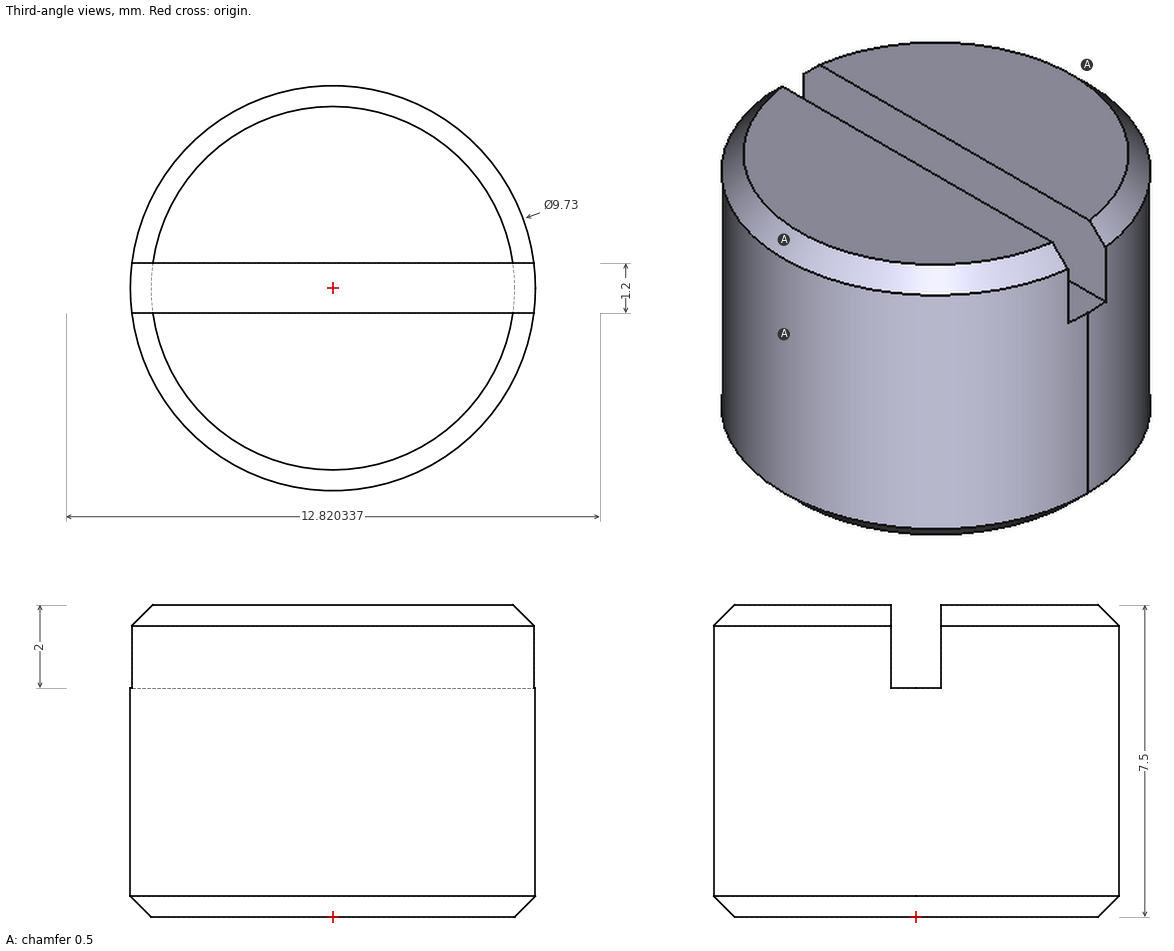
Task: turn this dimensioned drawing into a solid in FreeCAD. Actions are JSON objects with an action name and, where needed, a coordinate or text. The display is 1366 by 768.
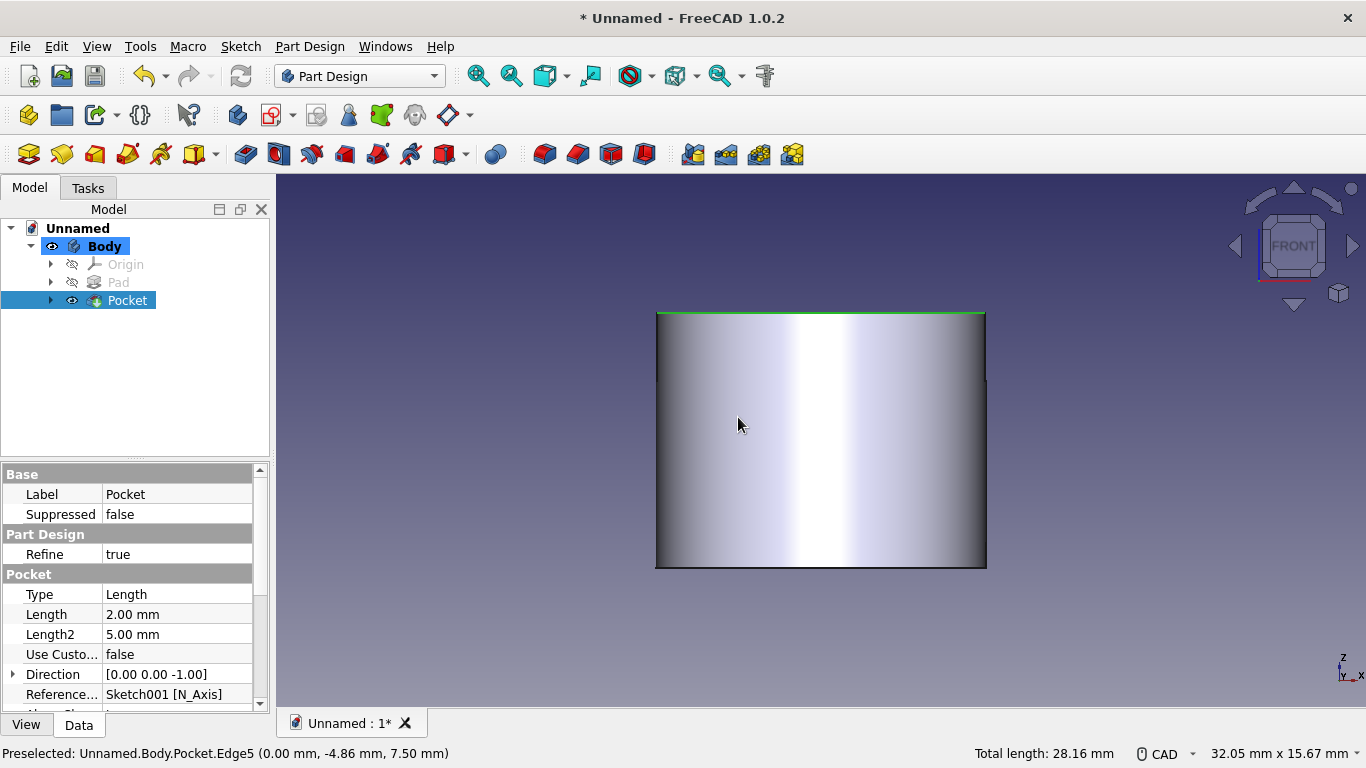
{"action": "key", "text": "3"}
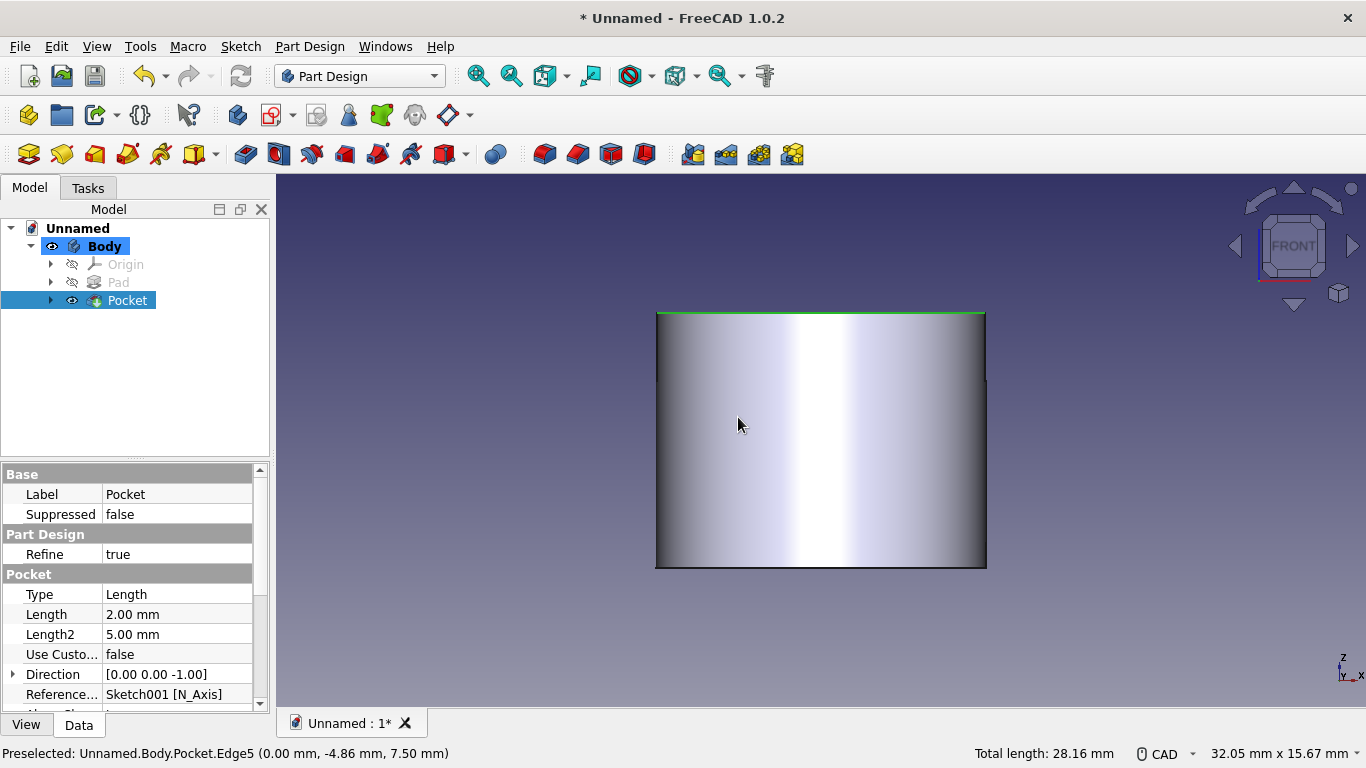
{"action": "left_click", "coordinate": [918, 567], "text": "ctrl"}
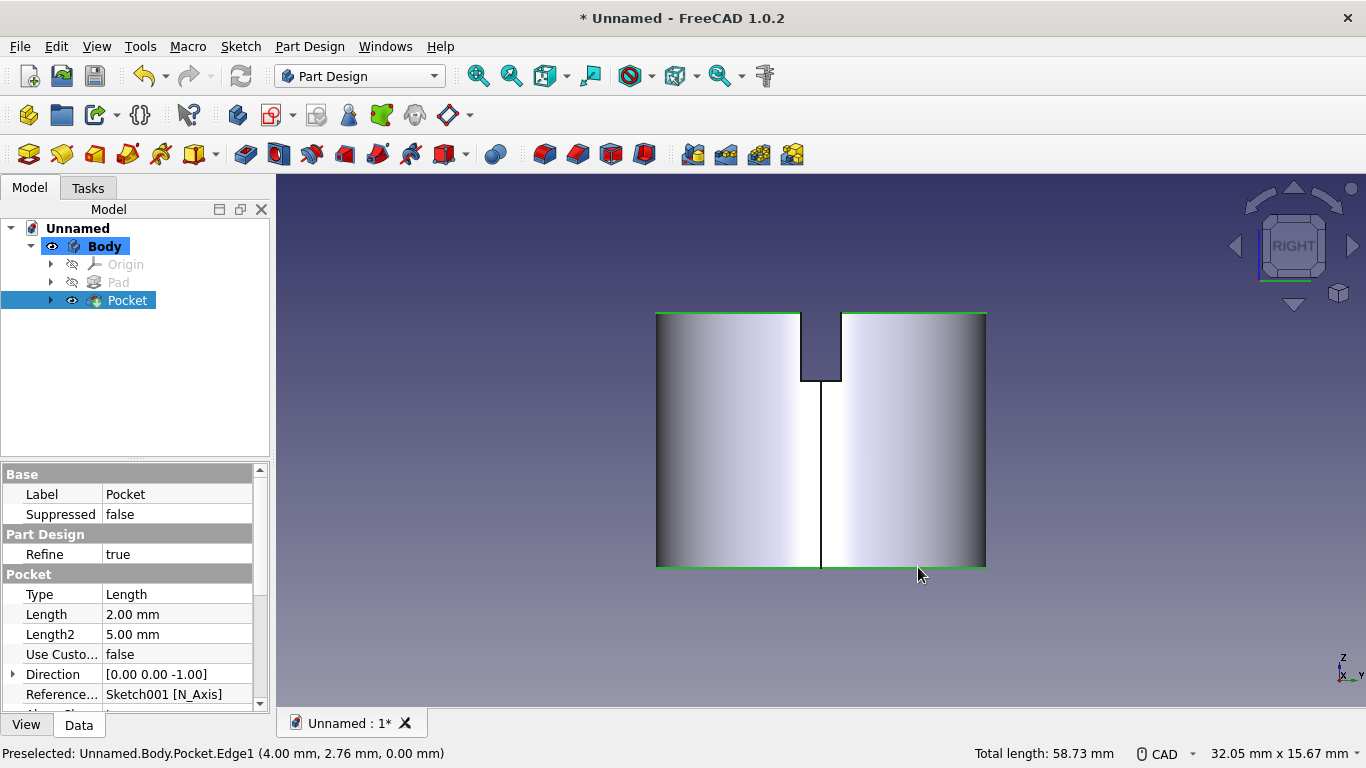
{"action": "left_click", "coordinate": [578, 154]}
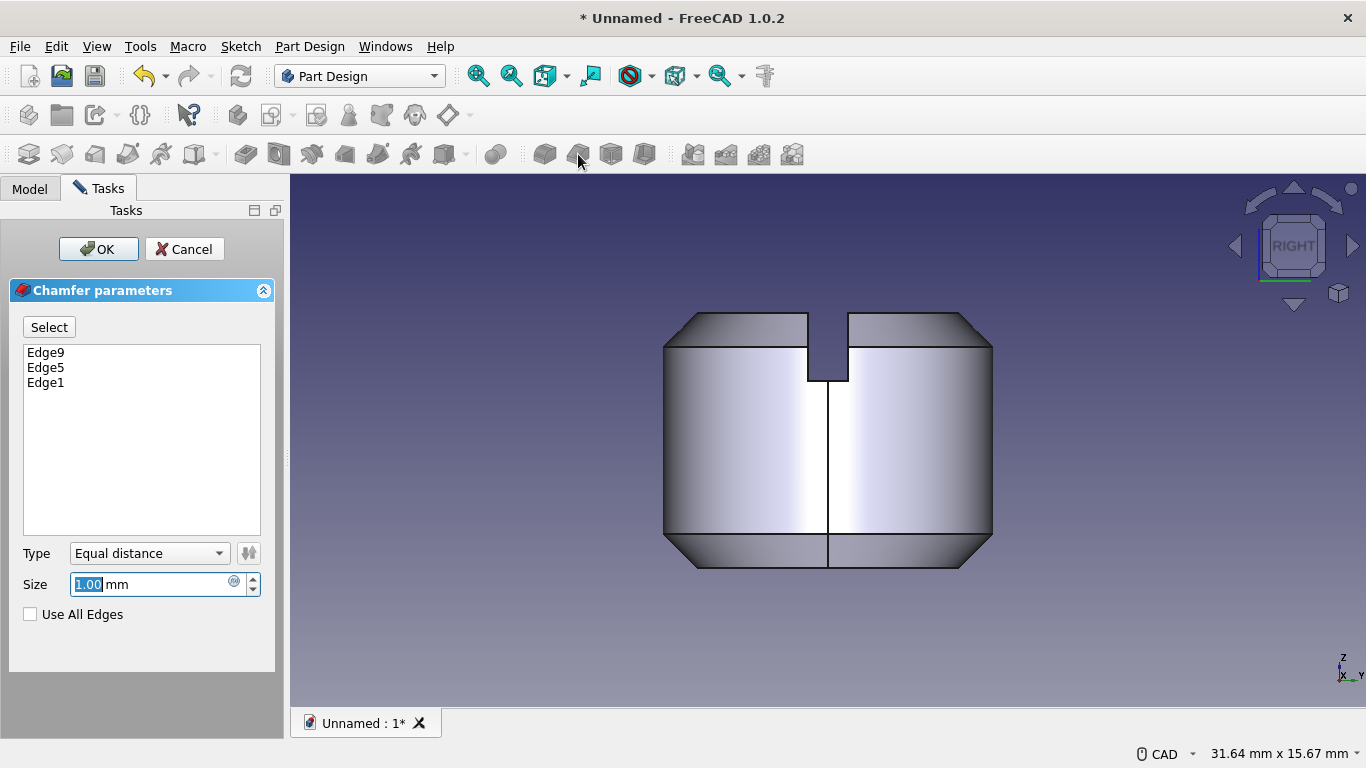
{"action": "type", "text": "0.5"}
{"action": "key", "text": "Tab"}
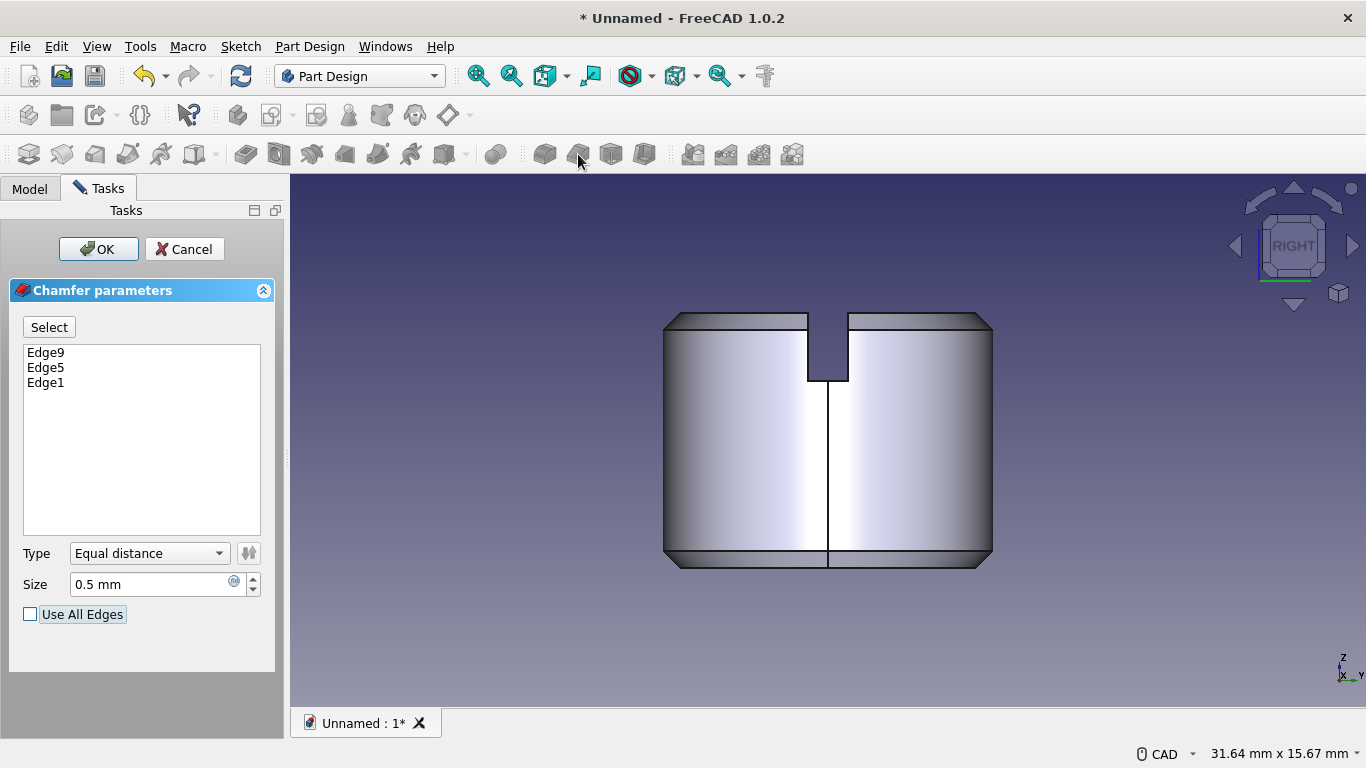
{"action": "left_click", "coordinate": [99, 249]}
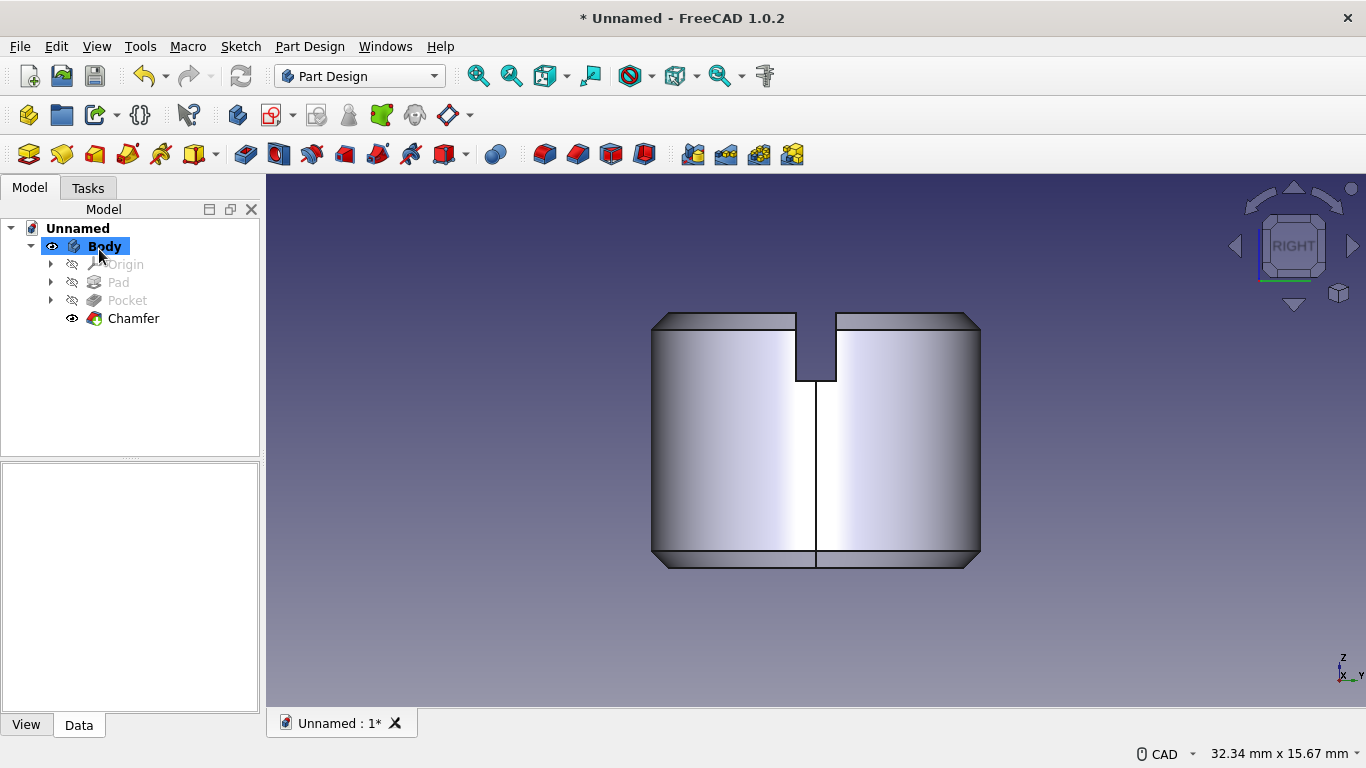
{"action": "key", "text": "0"}